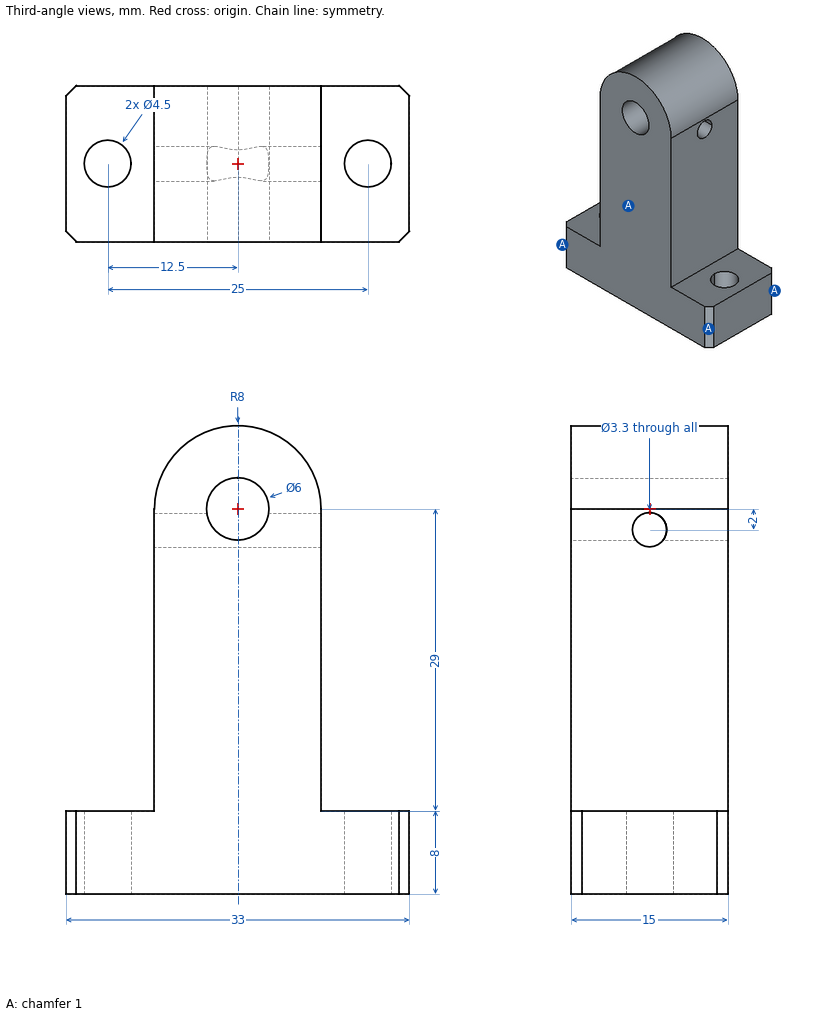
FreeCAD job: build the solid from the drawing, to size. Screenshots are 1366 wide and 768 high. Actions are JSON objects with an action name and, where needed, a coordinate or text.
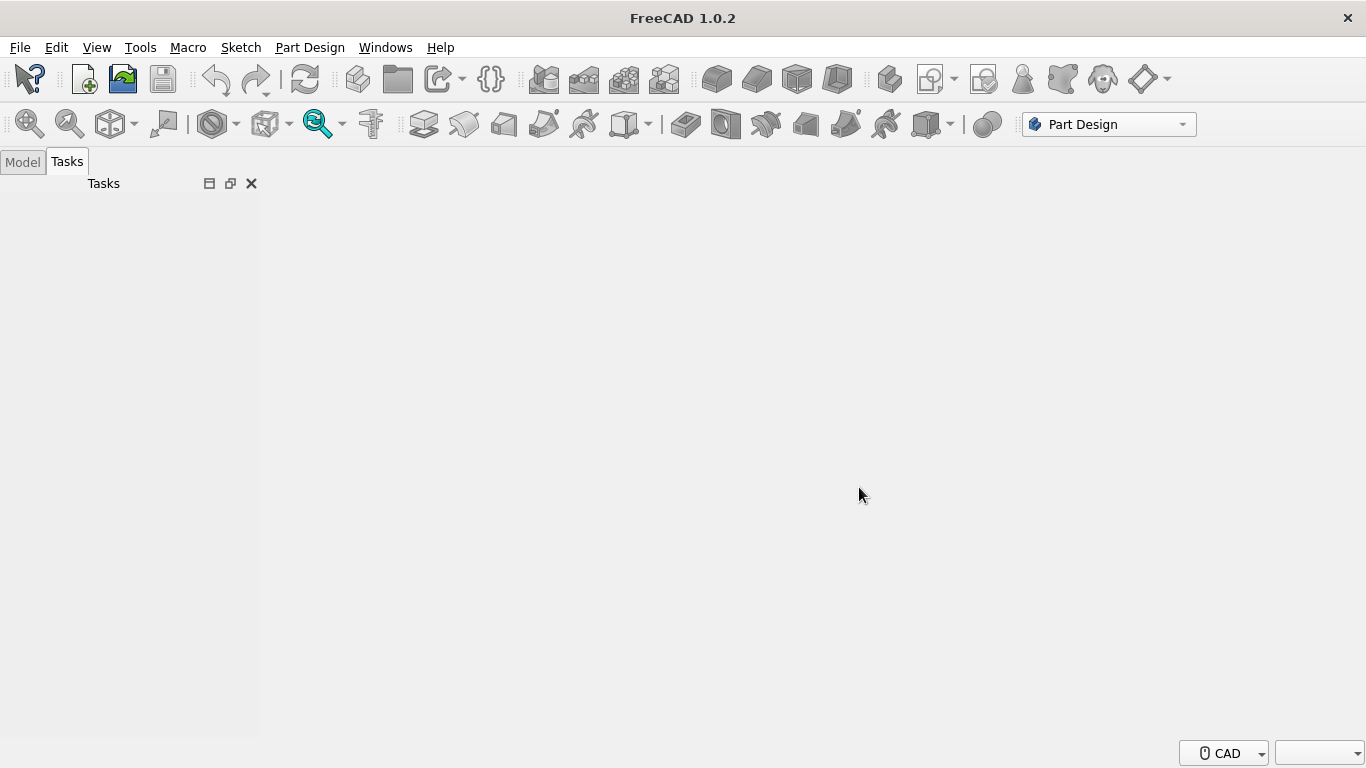
{"action": "key", "text": "ctrl+n"}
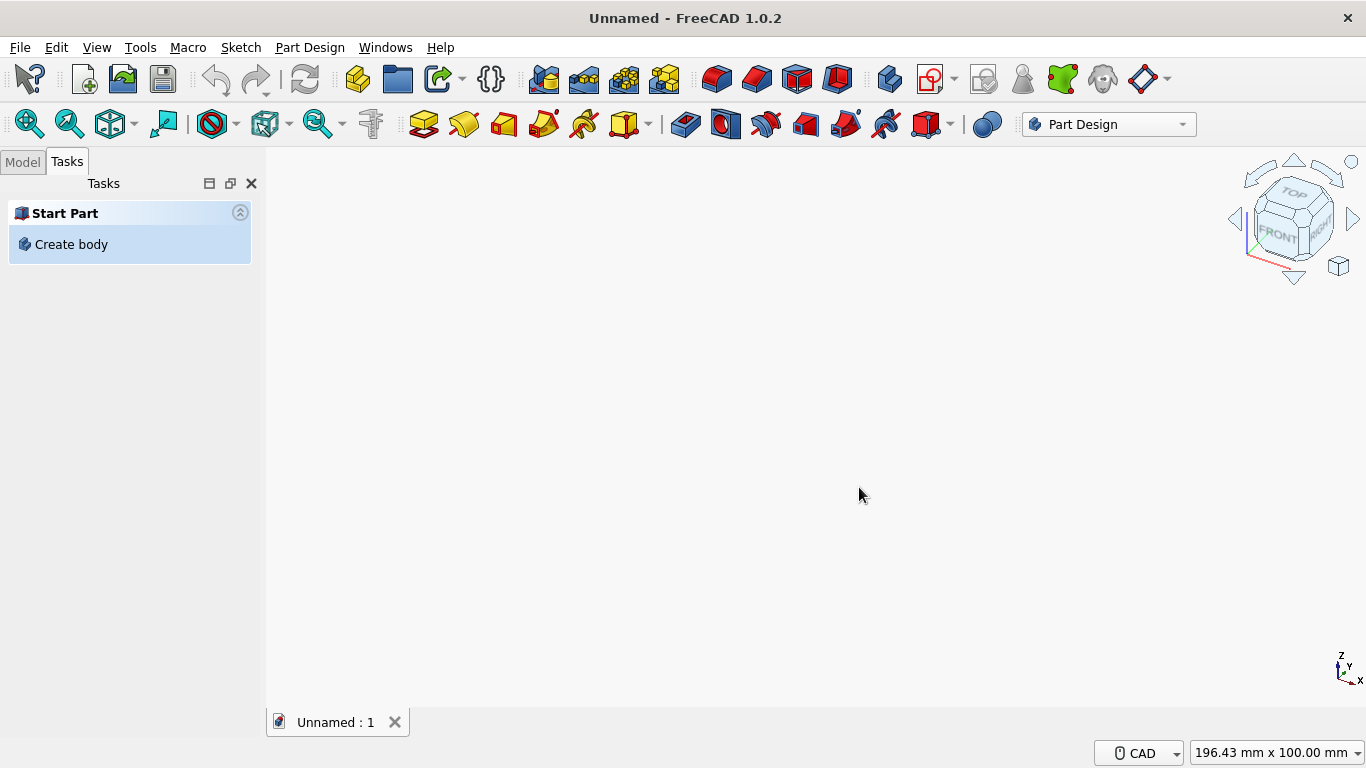
{"action": "left_click", "coordinate": [930, 80]}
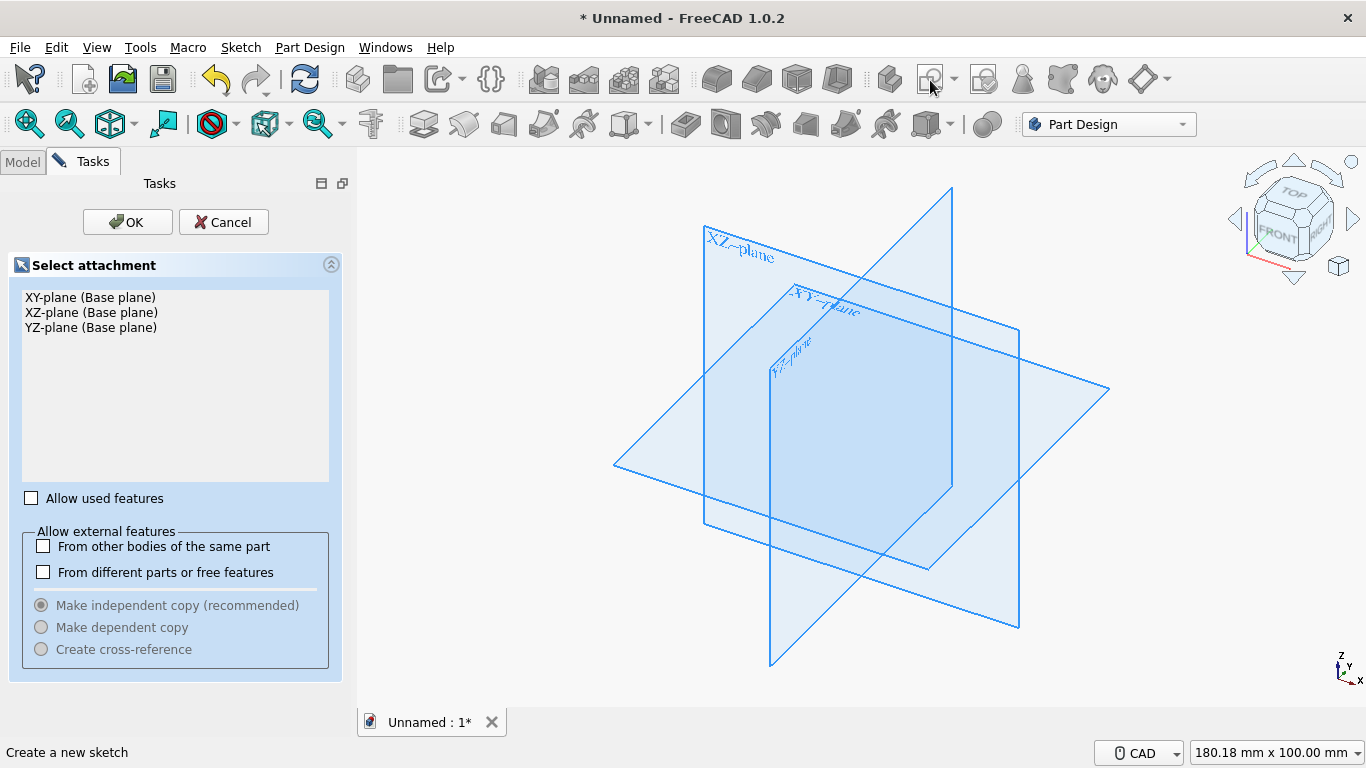
{"action": "left_click", "coordinate": [82, 312]}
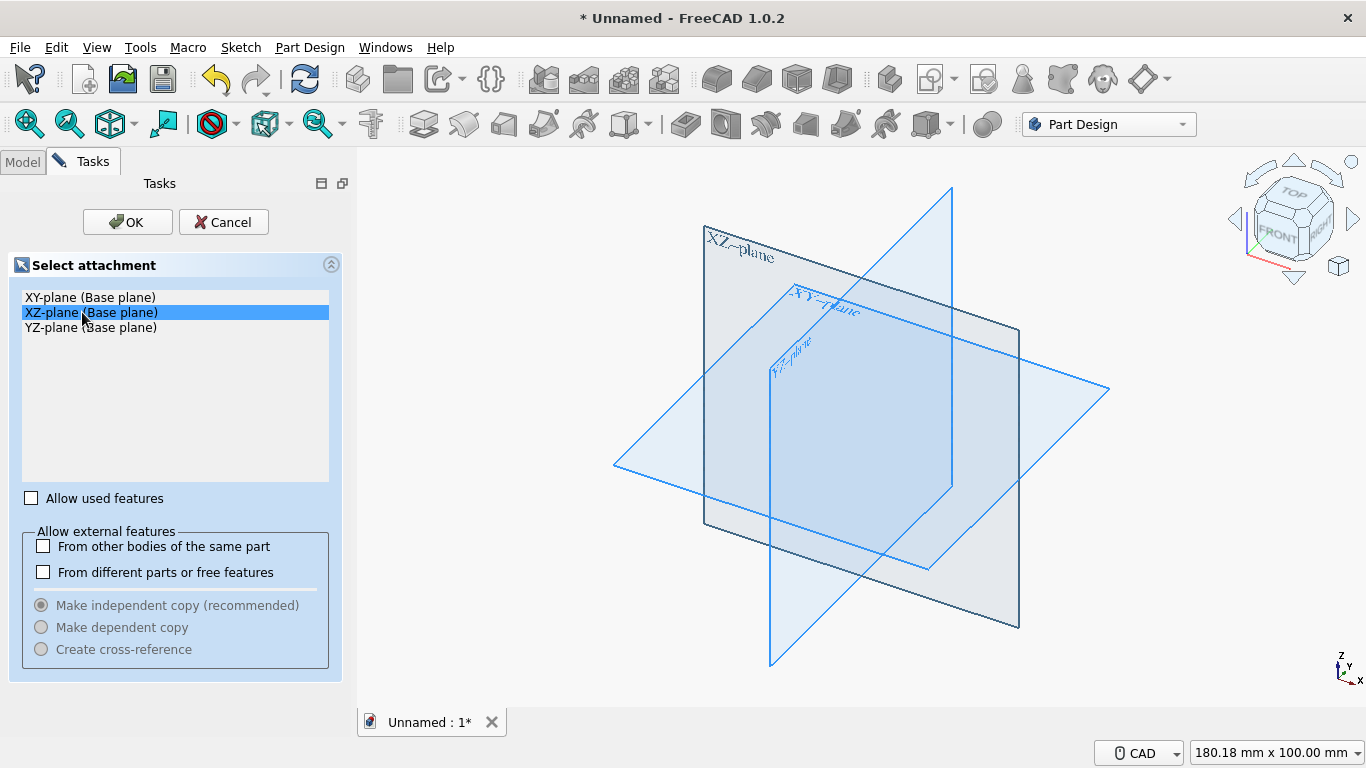
{"action": "left_click", "coordinate": [128, 222]}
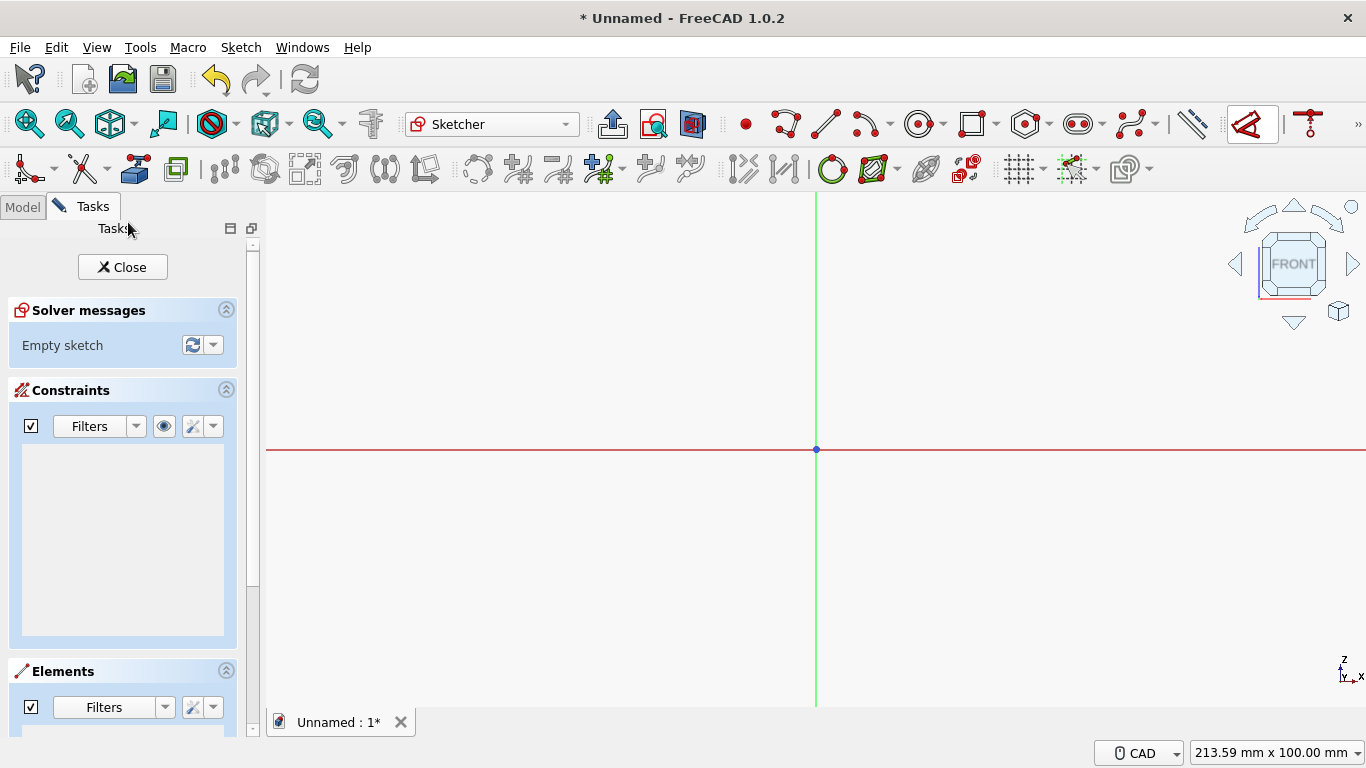
{"action": "scroll", "coordinate": [955, 676], "scroll_direction": "up", "scroll_amount": 2}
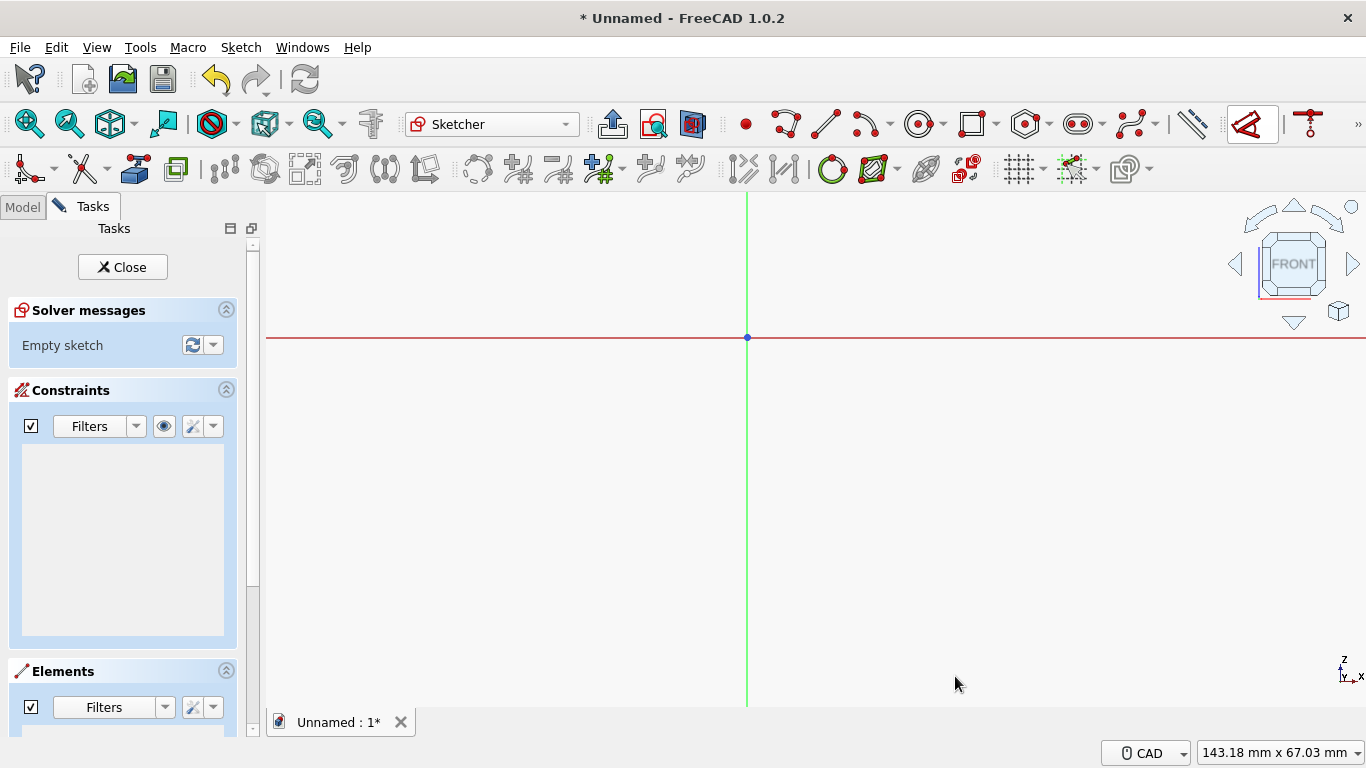
{"action": "left_click", "coordinate": [786, 124]}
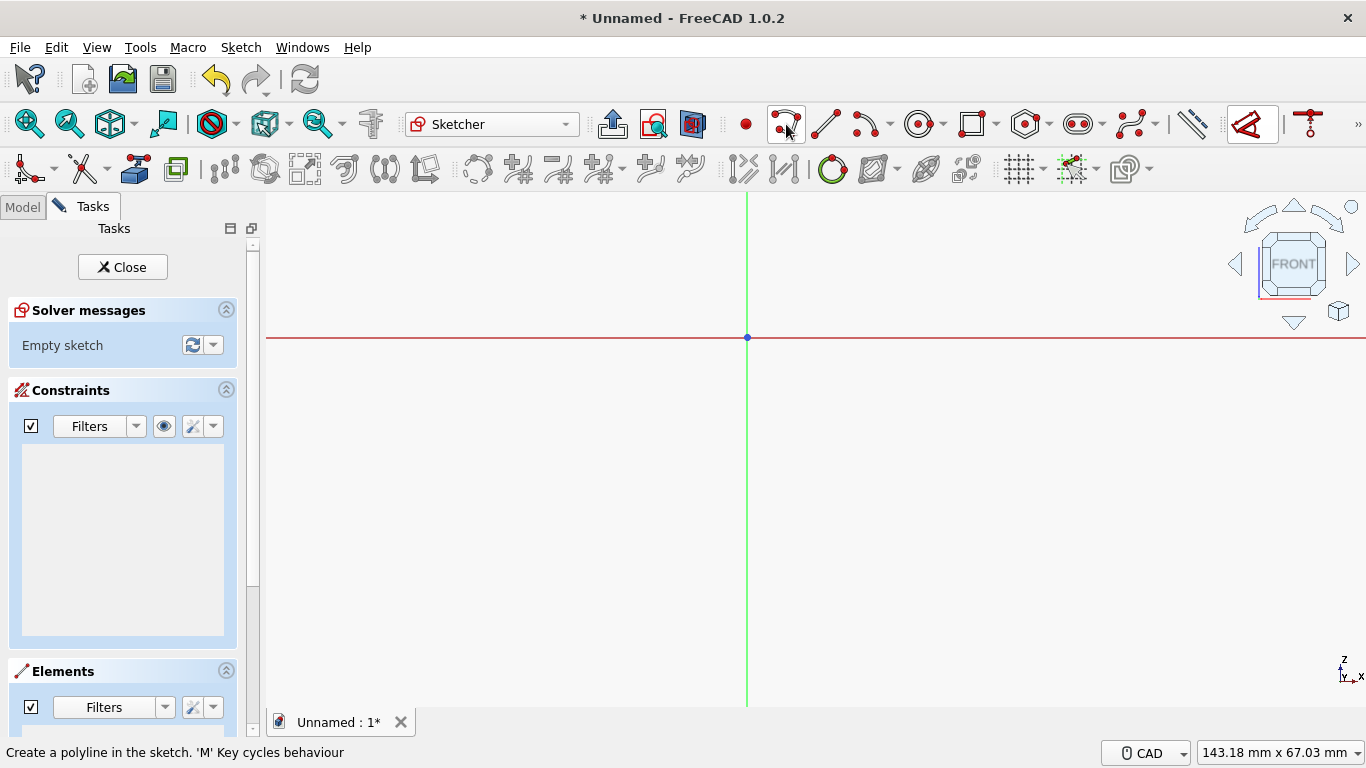
{"action": "left_click", "coordinate": [809, 338]}
{"action": "left_click", "coordinate": [809, 560]}
{"action": "left_click", "coordinate": [874, 560]}
{"action": "left_click", "coordinate": [874, 622]}
{"action": "left_click", "coordinate": [621, 622]}
{"action": "left_click", "coordinate": [621, 560]}
{"action": "left_click", "coordinate": [686, 560]}
{"action": "left_click", "coordinate": [686, 338]}
{"action": "right_click", "coordinate": [686, 338]}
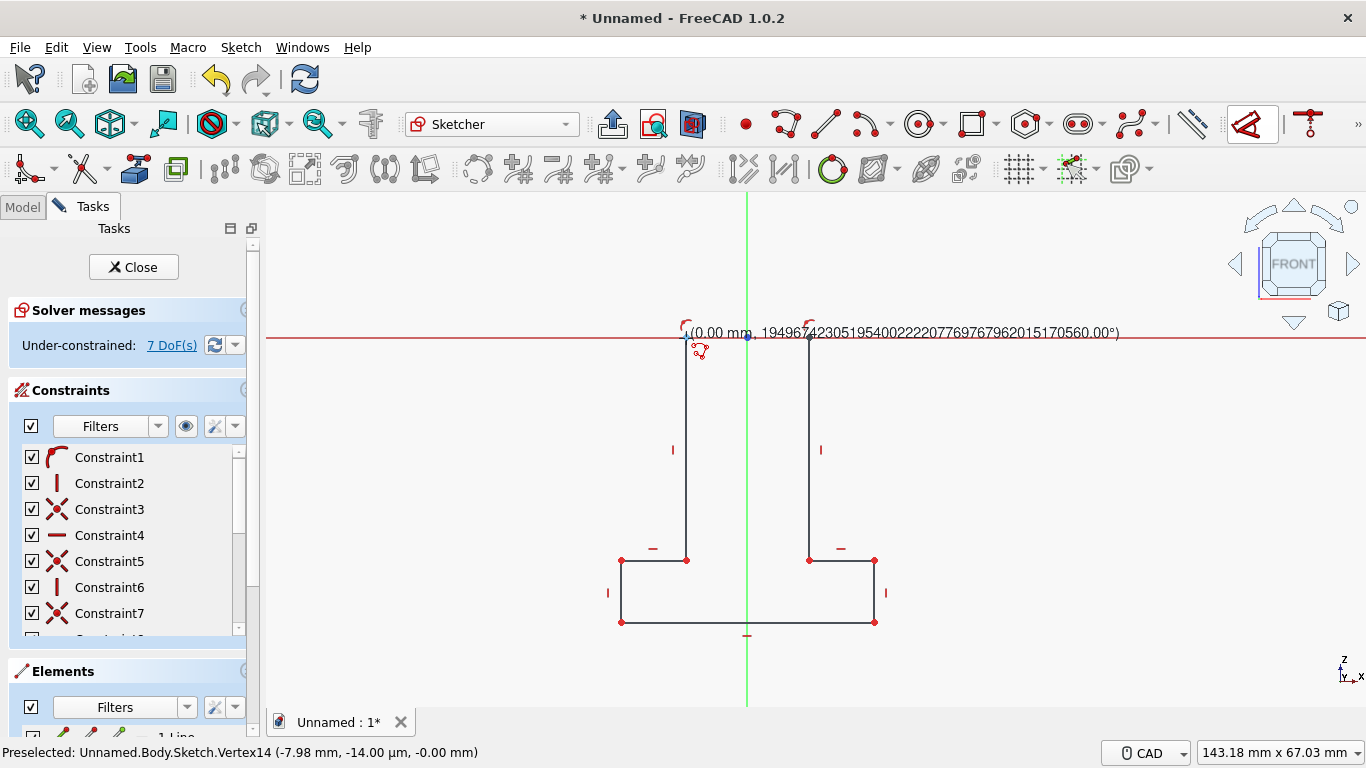
{"action": "key", "text": "g 3 a"}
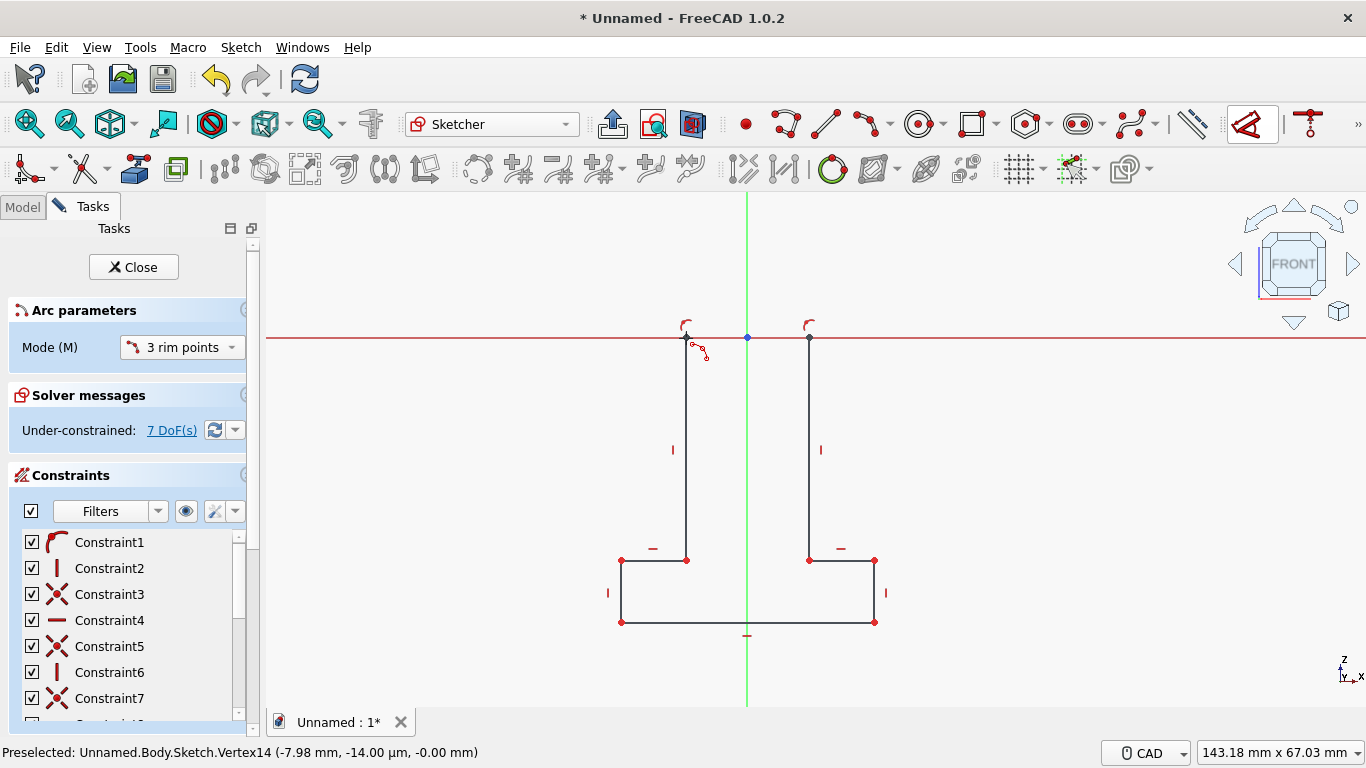
{"action": "left_click", "coordinate": [686, 338]}
{"action": "left_click", "coordinate": [809, 338]}
{"action": "left_click", "coordinate": [766, 279]}